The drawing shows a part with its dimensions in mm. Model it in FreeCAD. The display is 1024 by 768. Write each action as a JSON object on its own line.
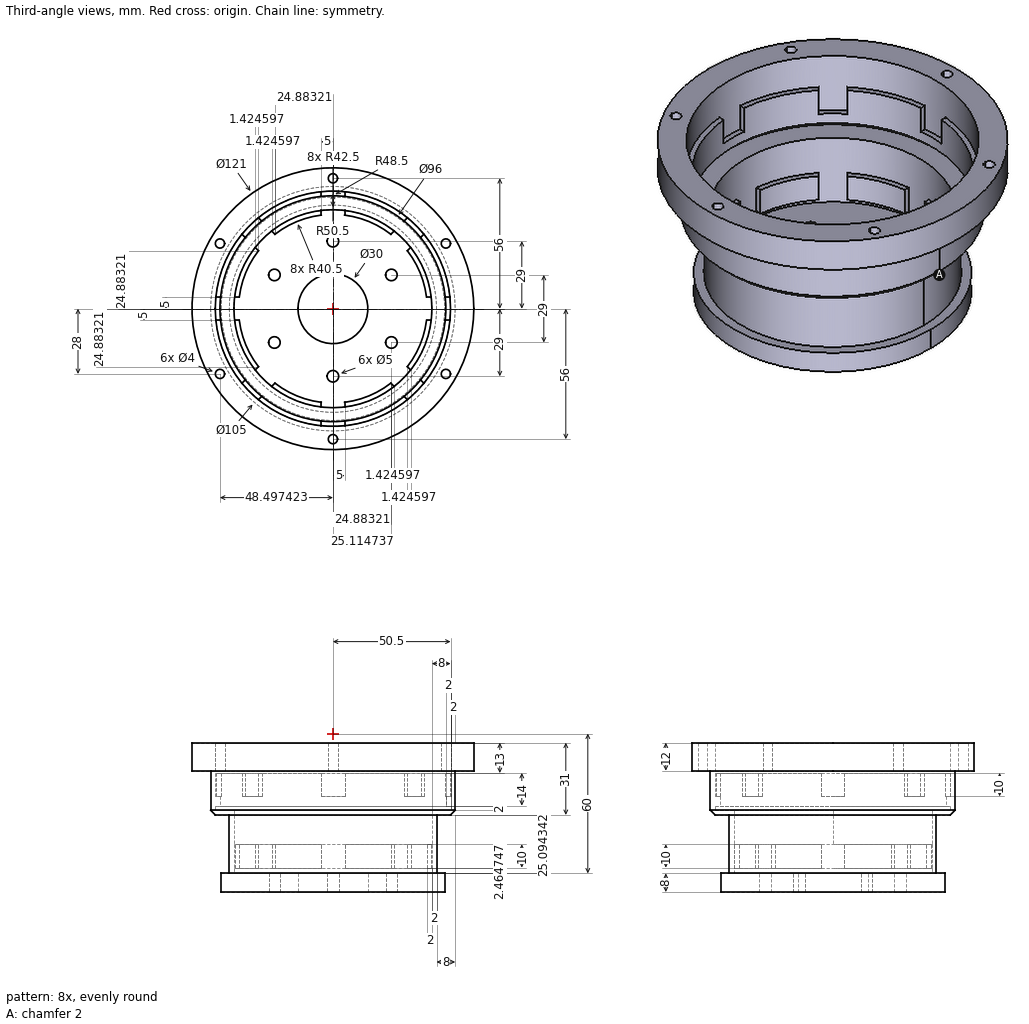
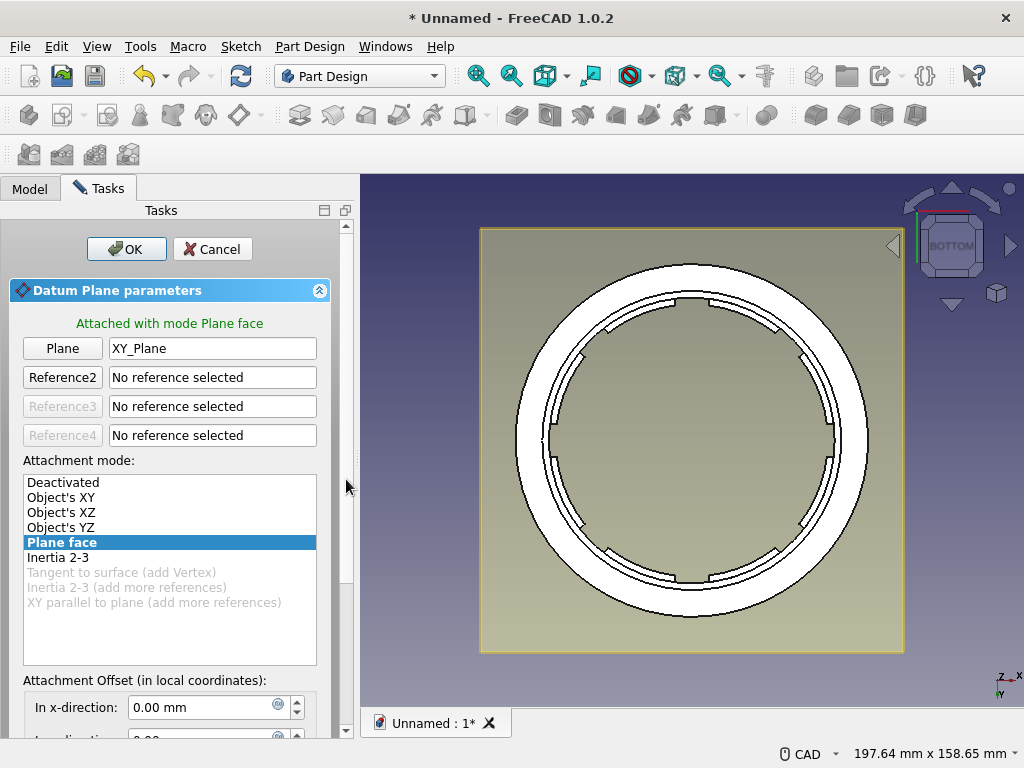
{"action": "left_click", "coordinate": [127, 249]}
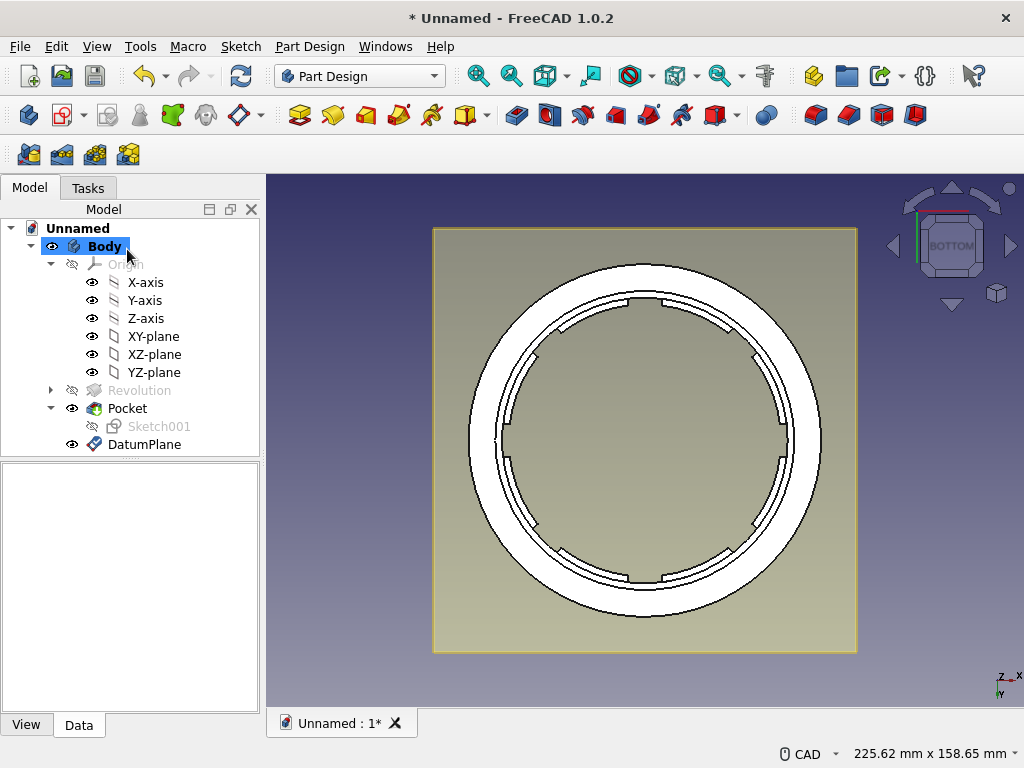
{"action": "left_click", "coordinate": [117, 444]}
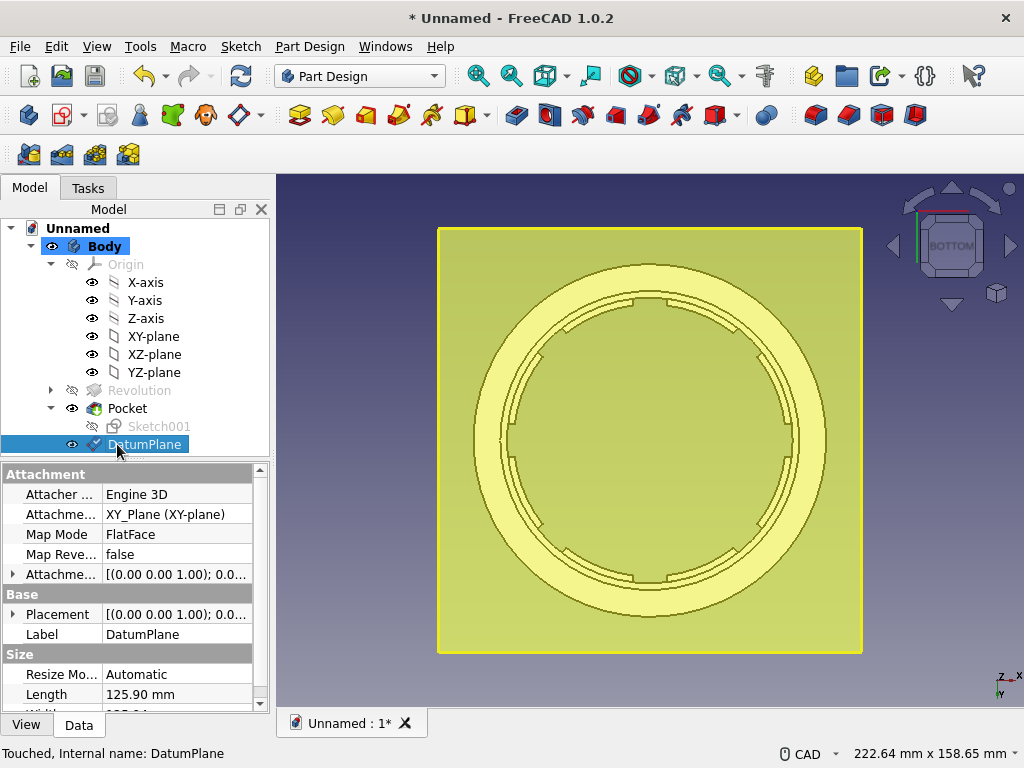
{"action": "left_click", "coordinate": [62, 116]}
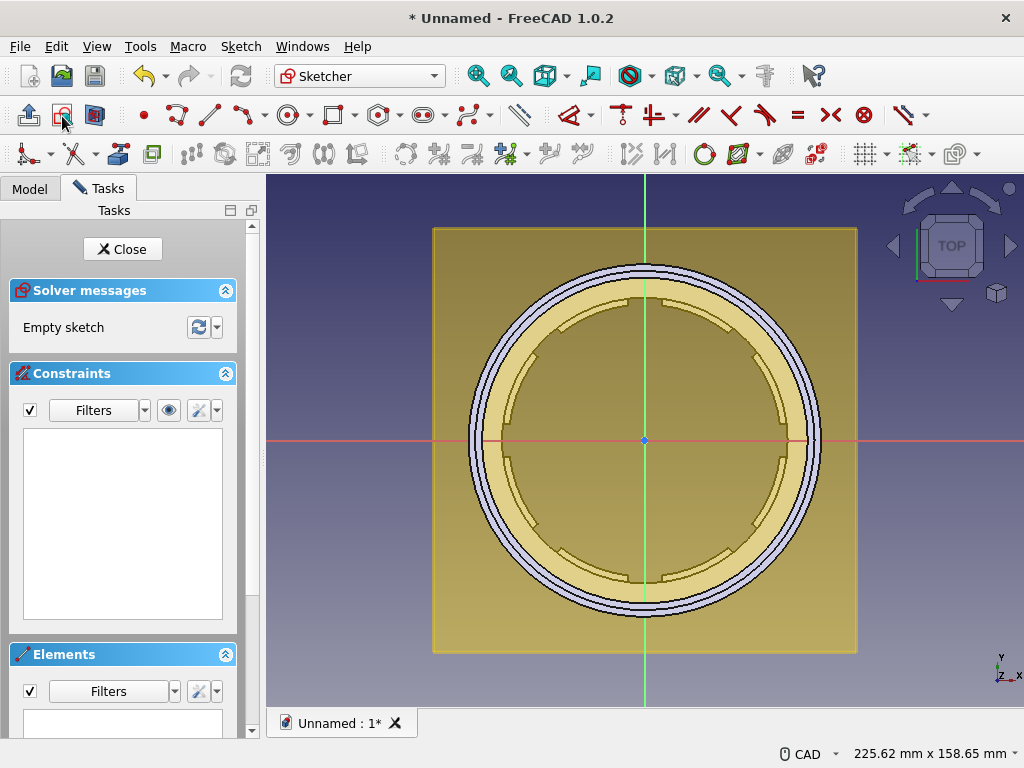
{"action": "key", "text": "q s"}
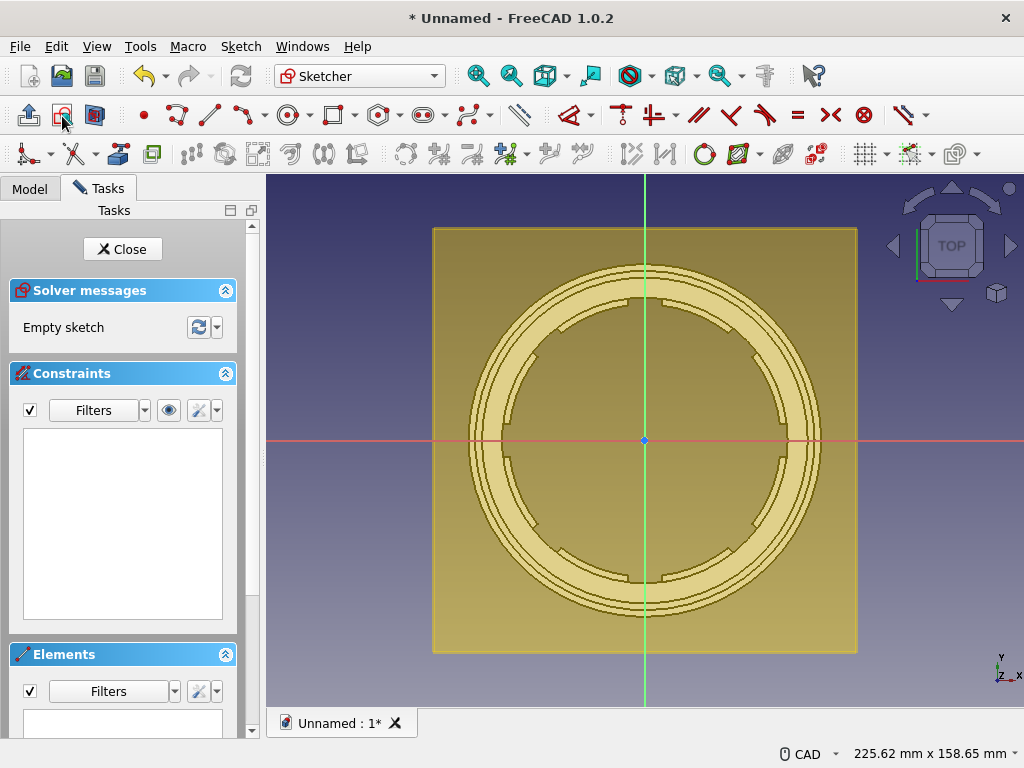
{"action": "scroll", "coordinate": [652, 258], "scroll_direction": "up", "scroll_amount": 12}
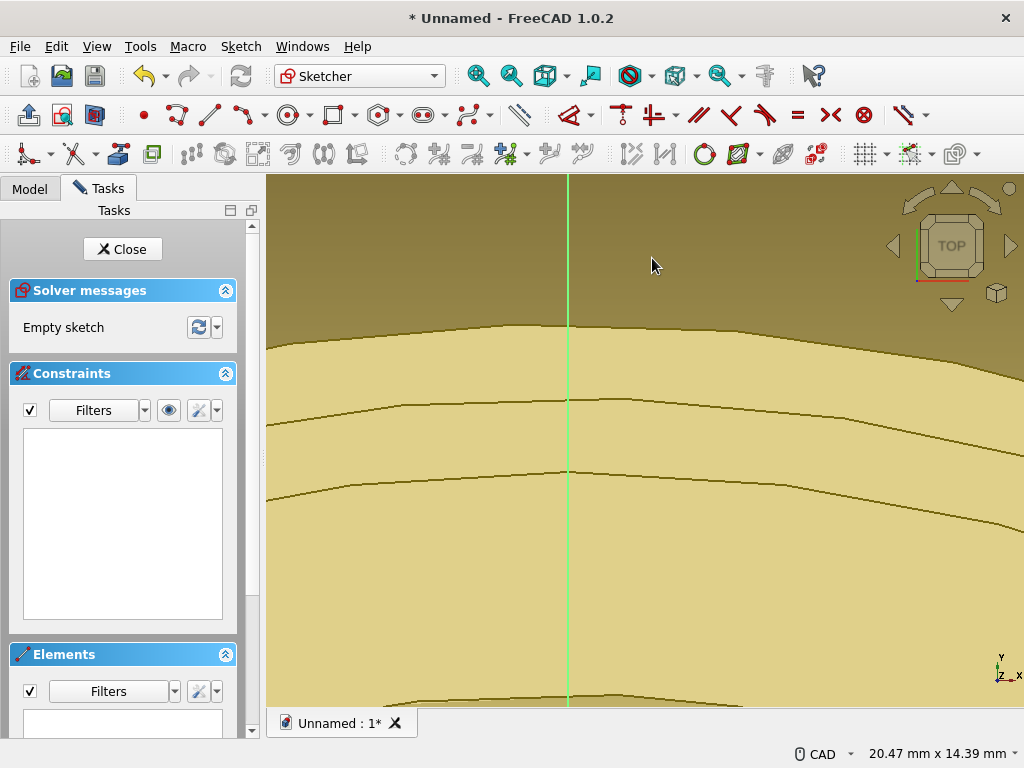
{"action": "left_click", "coordinate": [210, 116]}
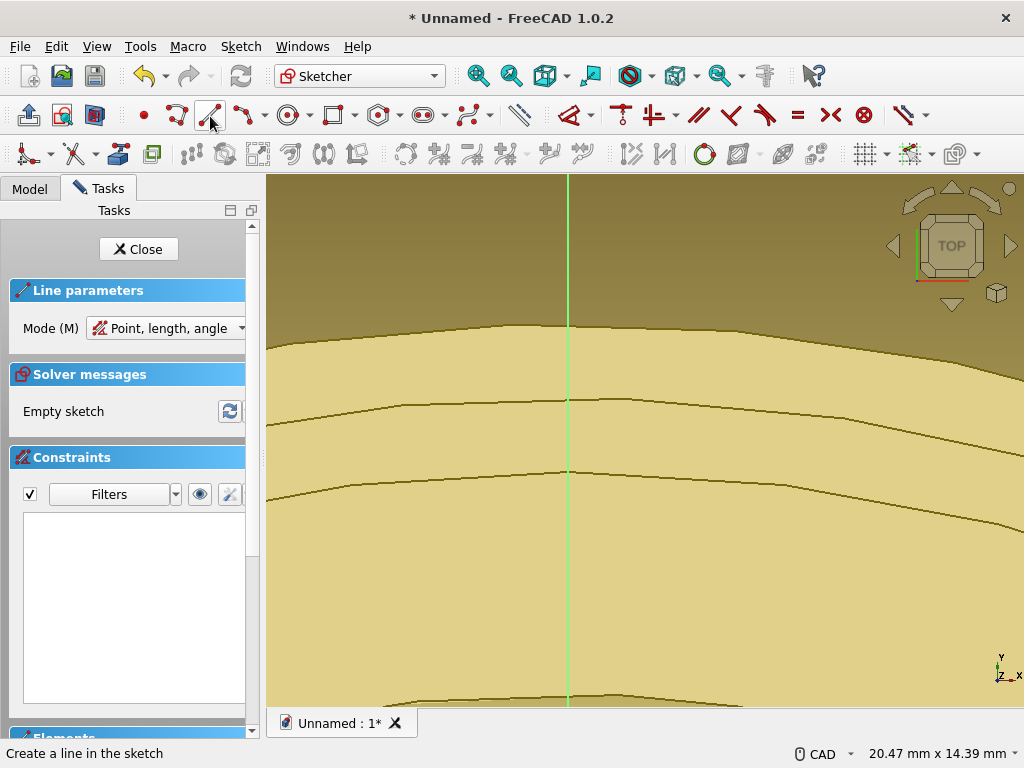
{"action": "left_click", "coordinate": [383, 407]}
{"action": "left_click", "coordinate": [383, 482]}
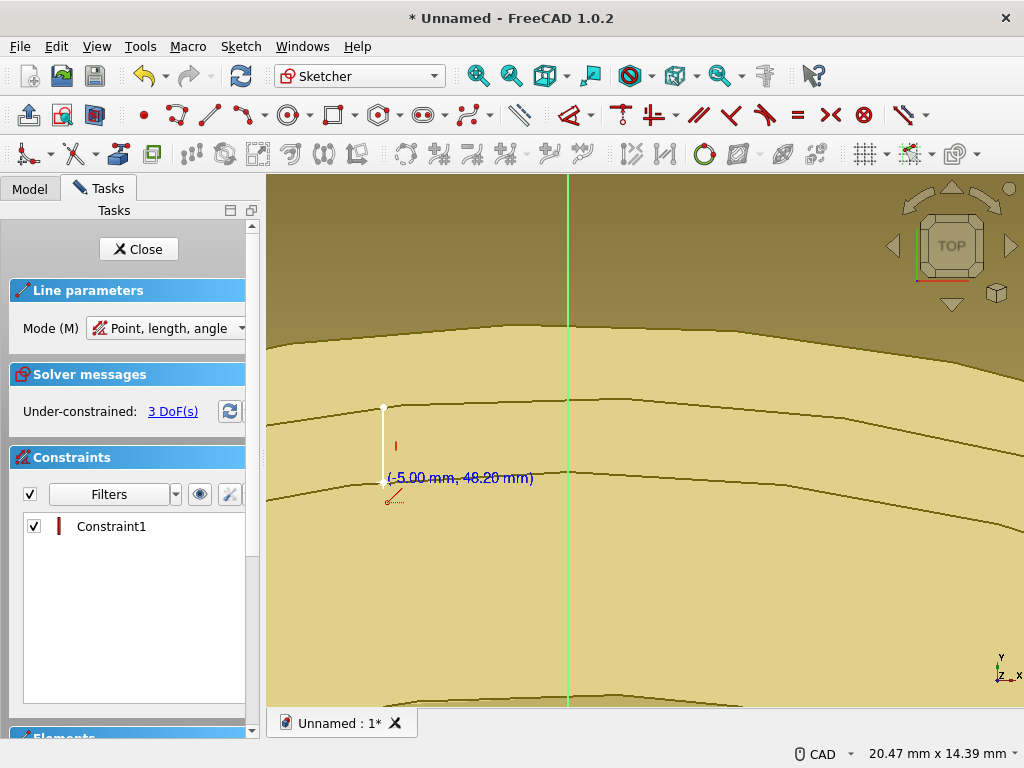
{"action": "left_click", "coordinate": [753, 482]}
{"action": "left_click", "coordinate": [753, 407]}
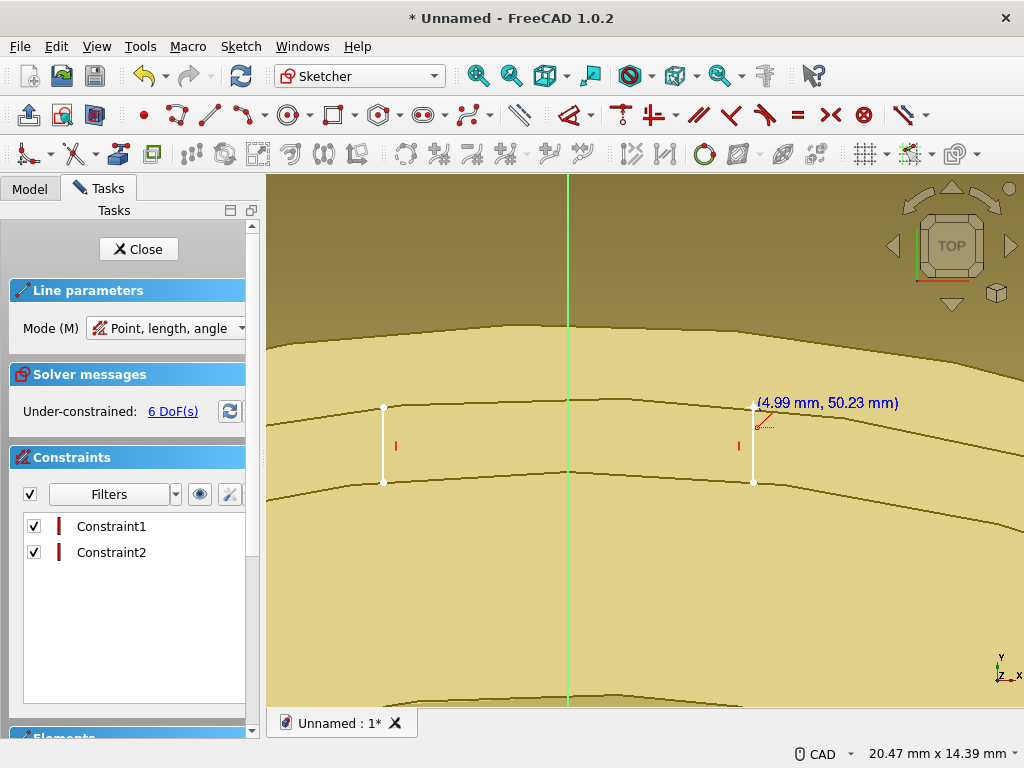
{"action": "key", "text": "g 3 a"}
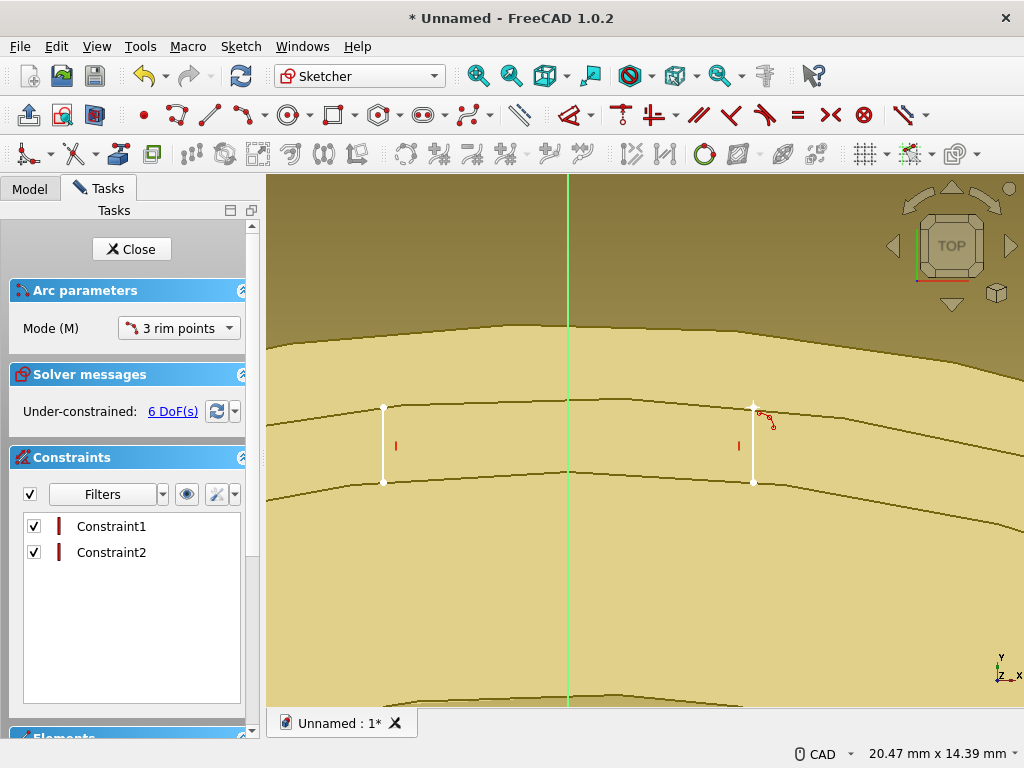
{"action": "left_click", "coordinate": [383, 483]}
{"action": "left_click", "coordinate": [753, 483]}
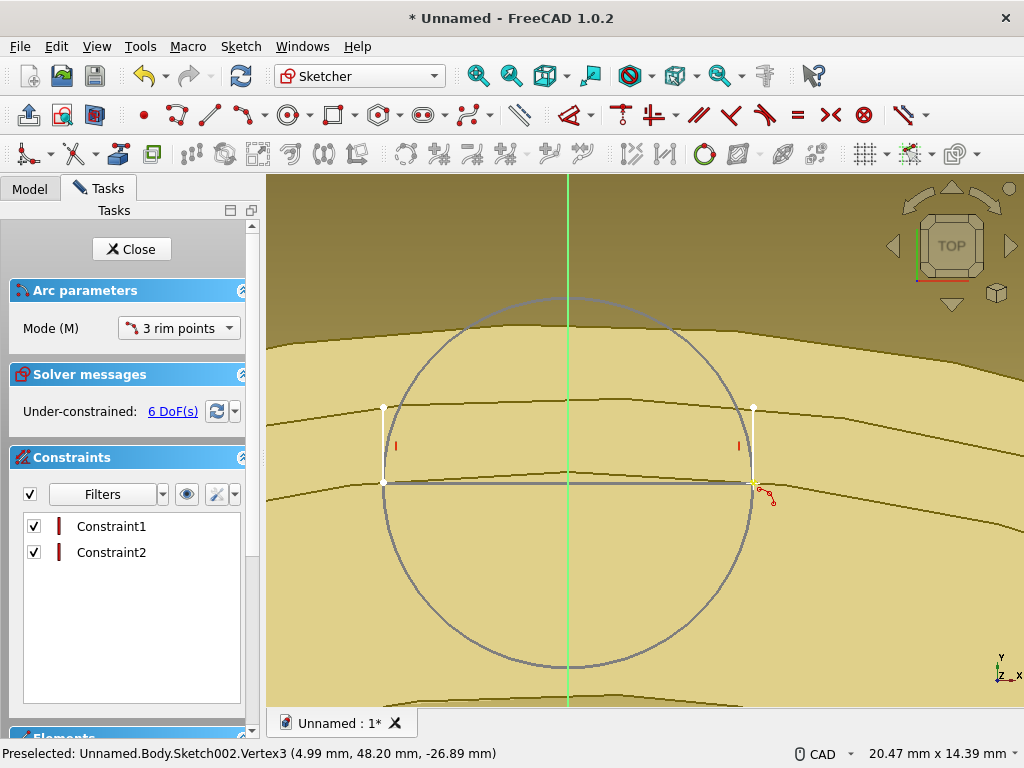
{"action": "scroll", "coordinate": [605, 472], "scroll_direction": "up", "scroll_amount": 3}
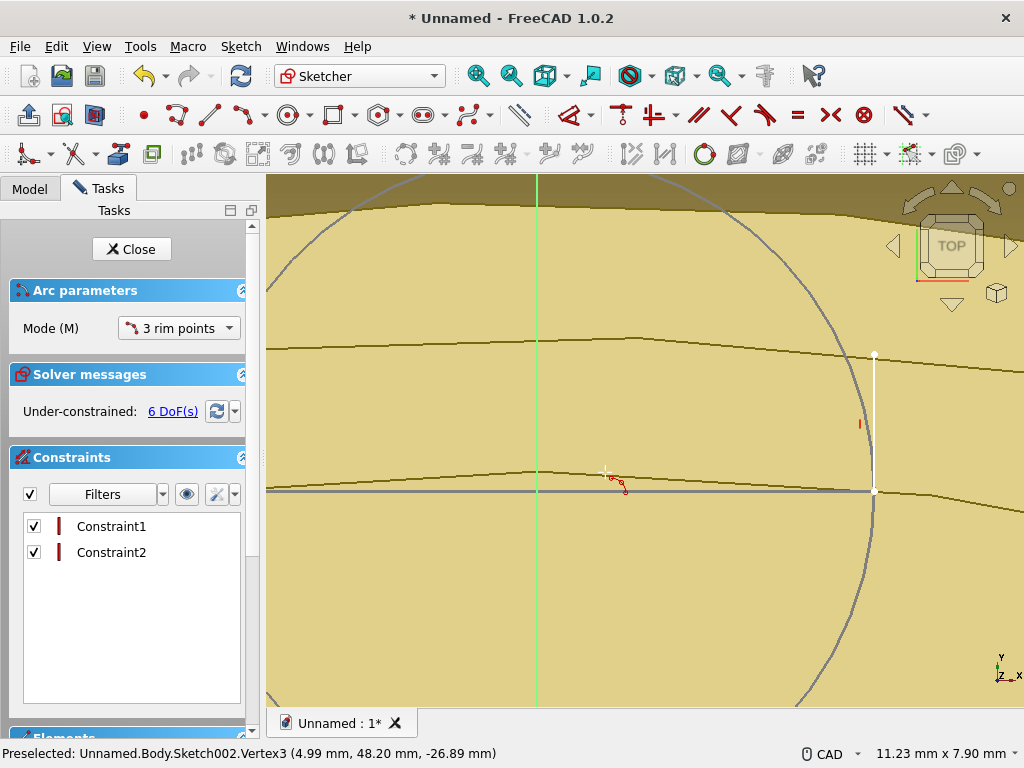
{"action": "left_click", "coordinate": [605, 472]}